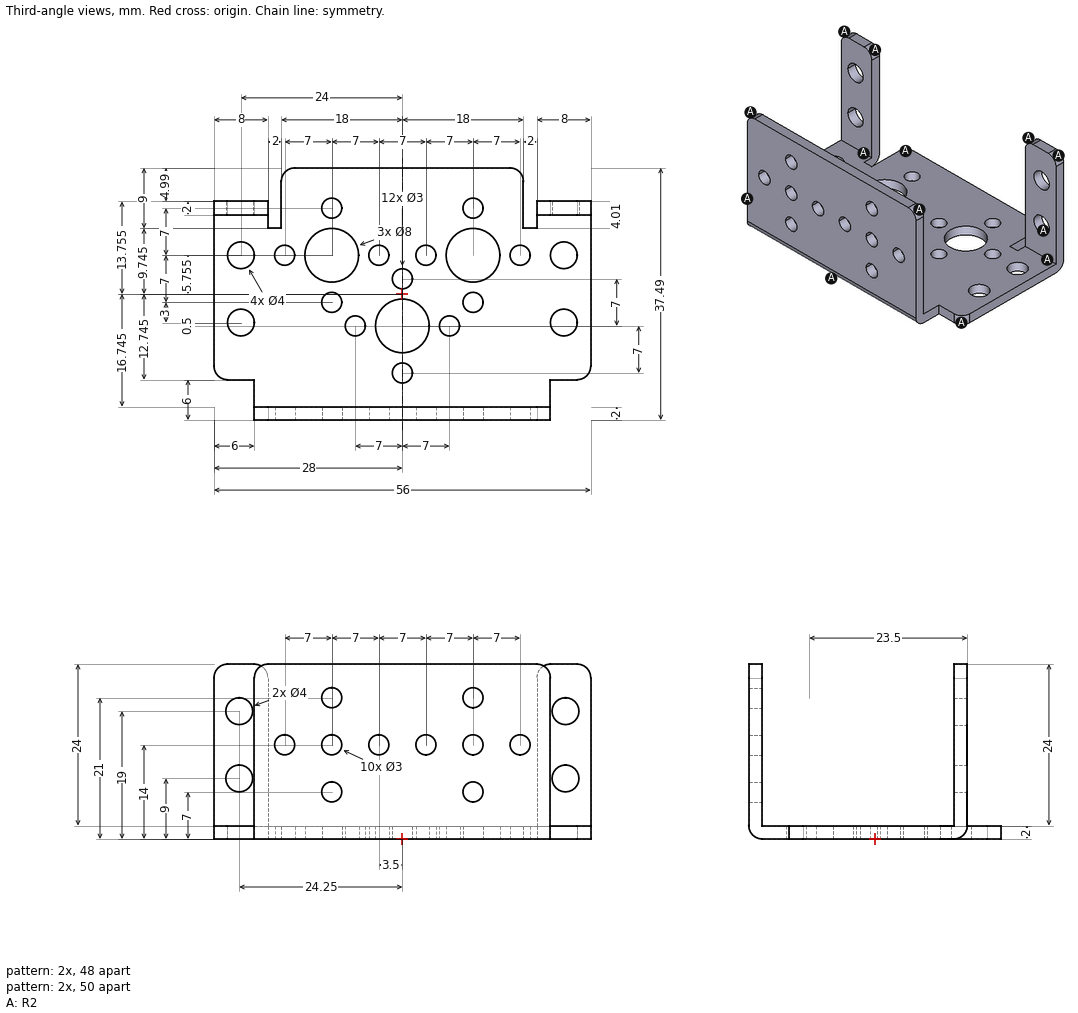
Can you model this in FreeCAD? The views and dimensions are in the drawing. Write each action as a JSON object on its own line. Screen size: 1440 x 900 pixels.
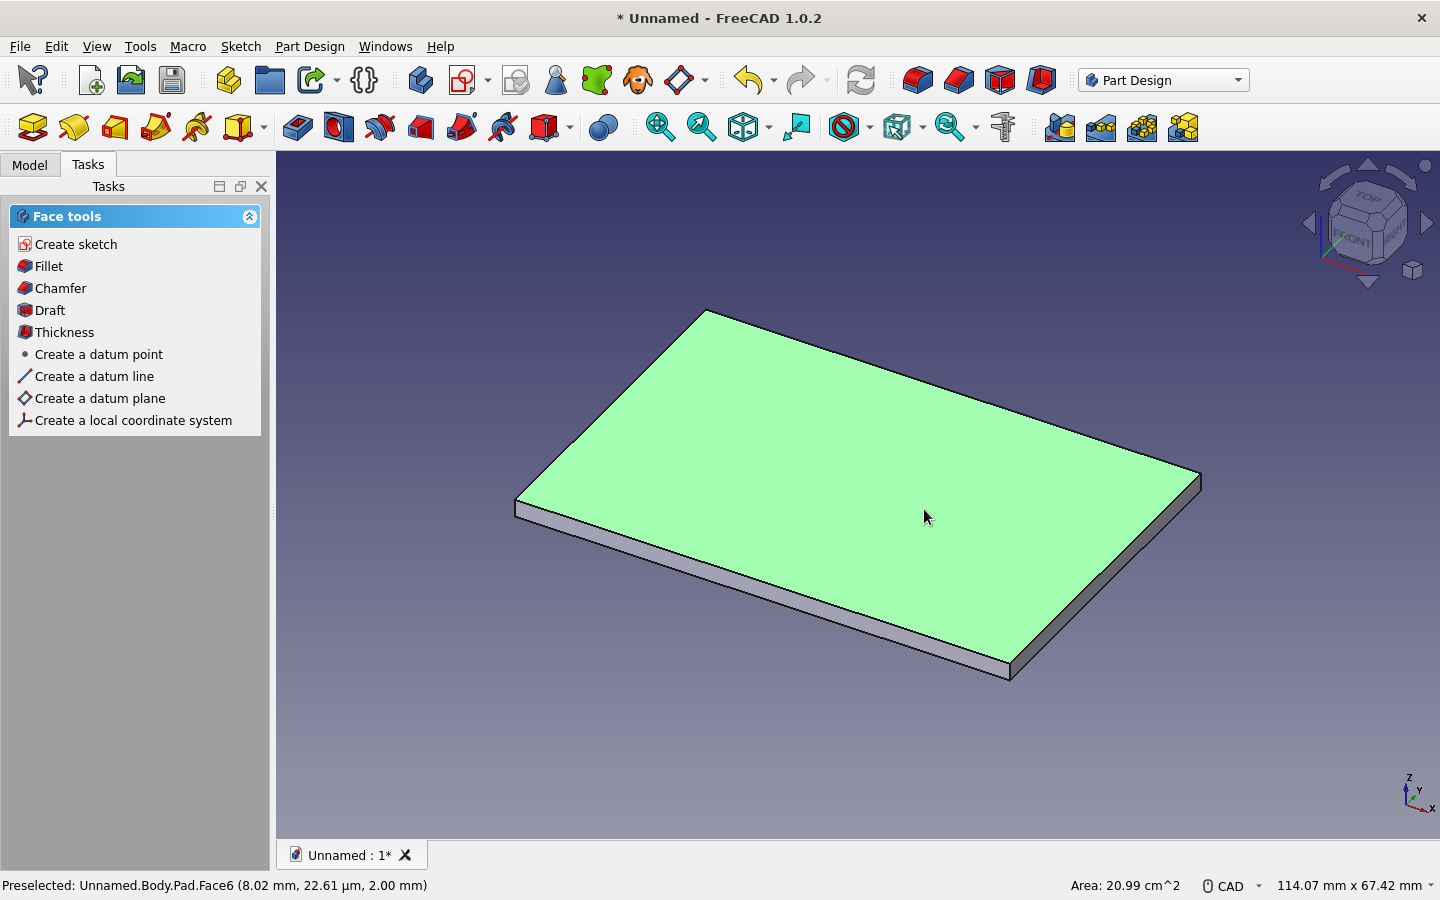
{"action": "left_click", "coordinate": [462, 80]}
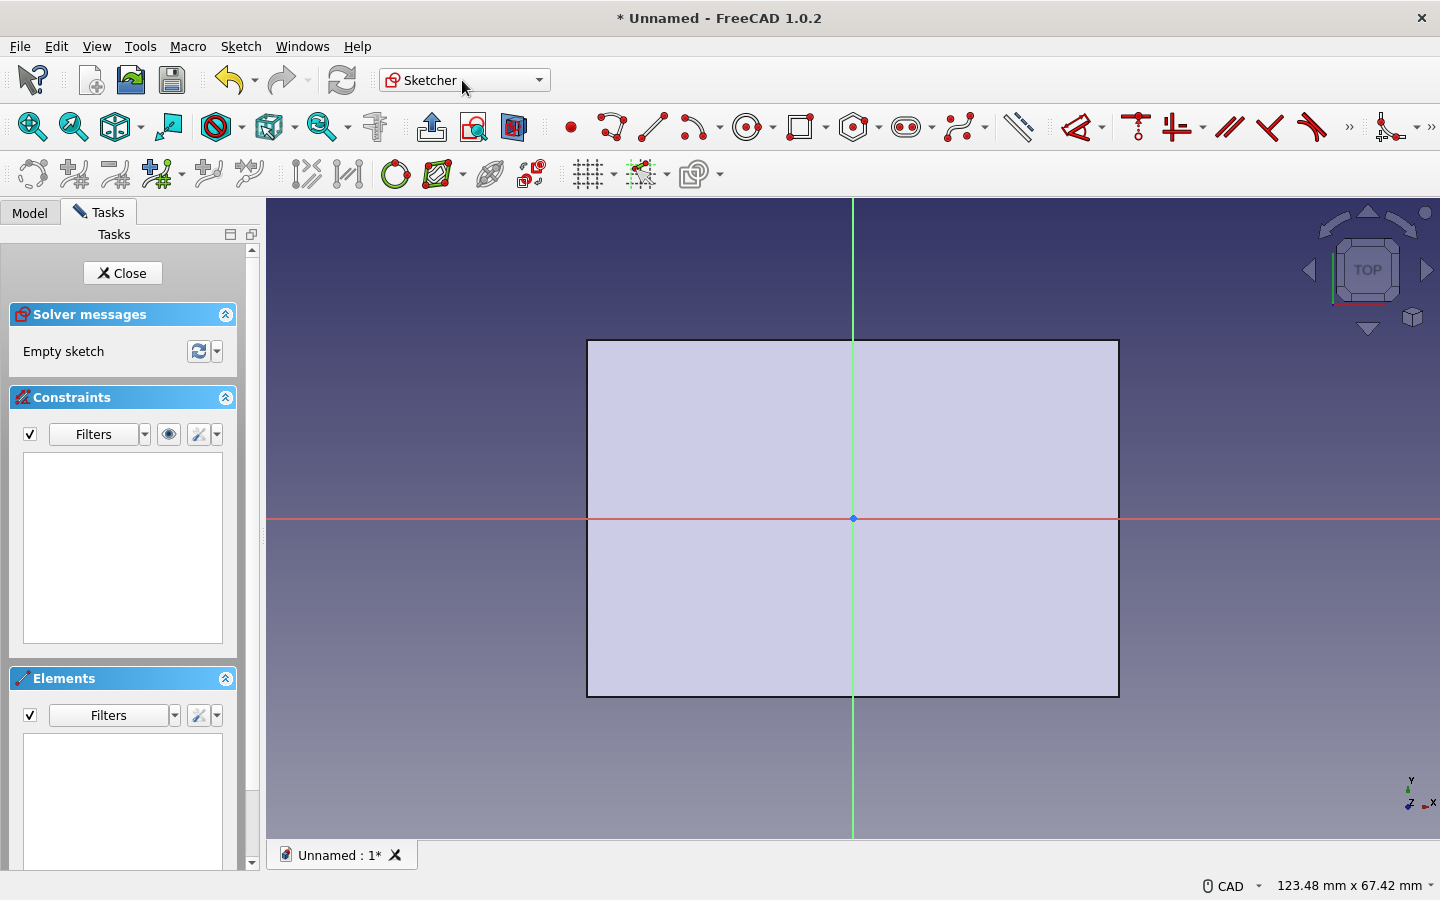
{"action": "key", "text": "g r"}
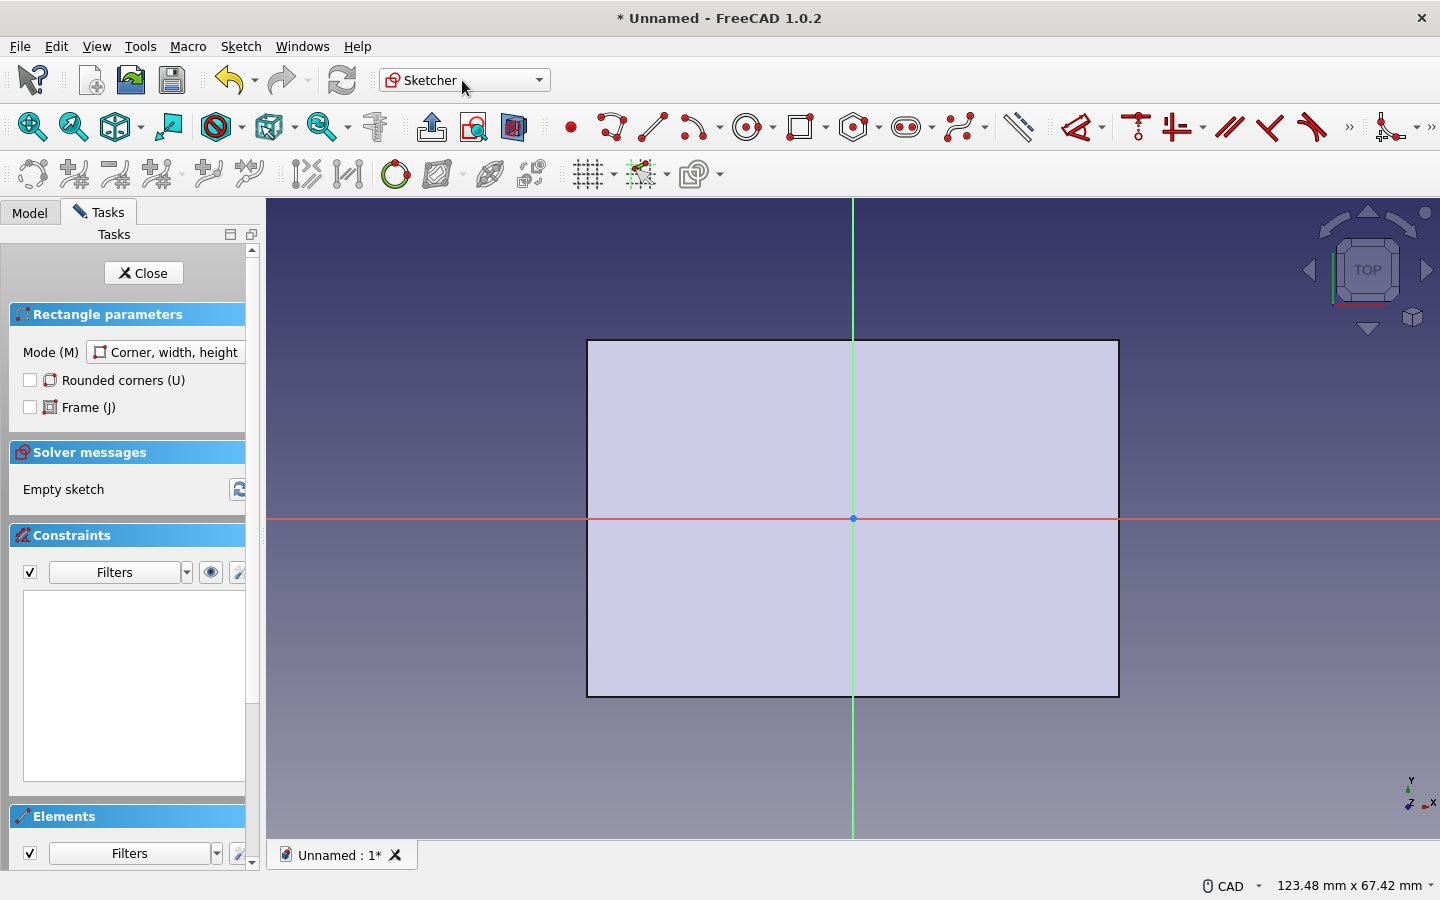
{"action": "left_click", "coordinate": [587, 678]}
{"action": "mouse_move", "coordinate": [1119, 697]}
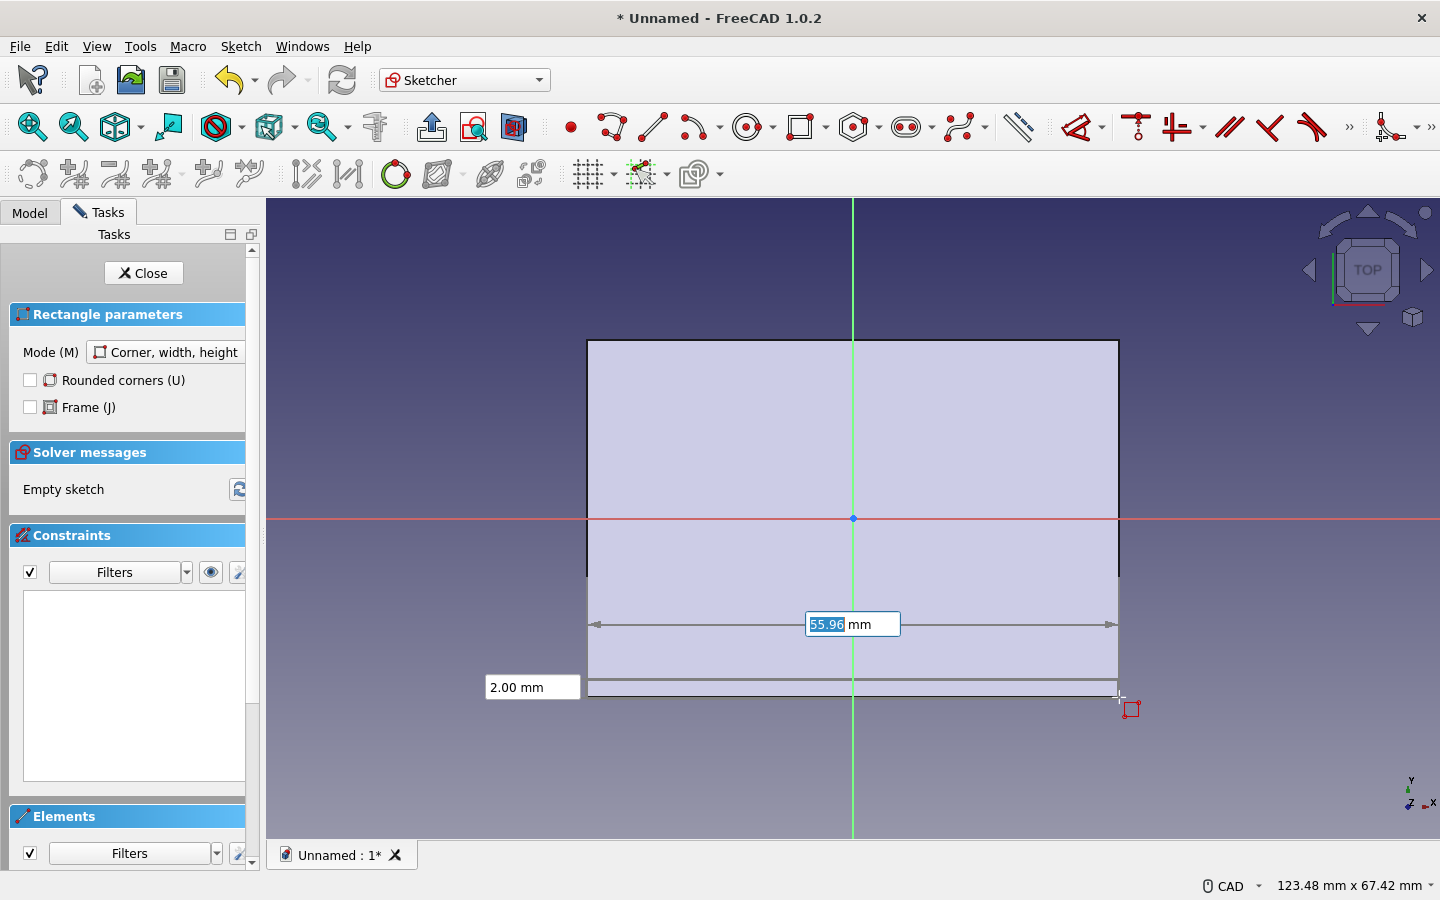
{"action": "type", "text": "56"}
{"action": "key", "text": "Tab"}
{"action": "type", "text": "2"}
{"action": "key", "text": "Return"}
{"action": "key", "text": "Escape"}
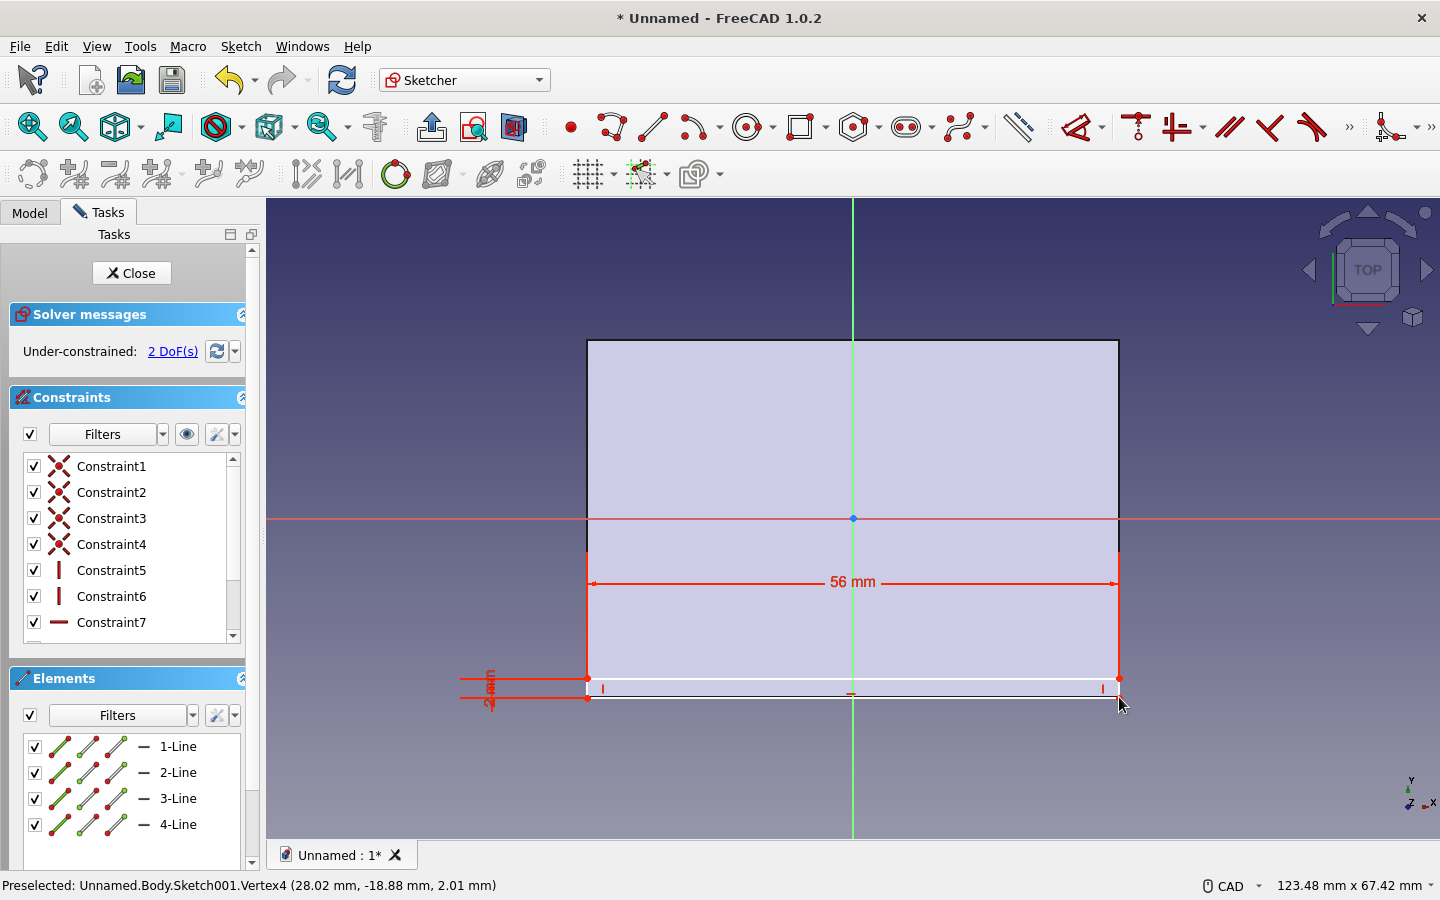
{"action": "left_click", "coordinate": [587, 679]}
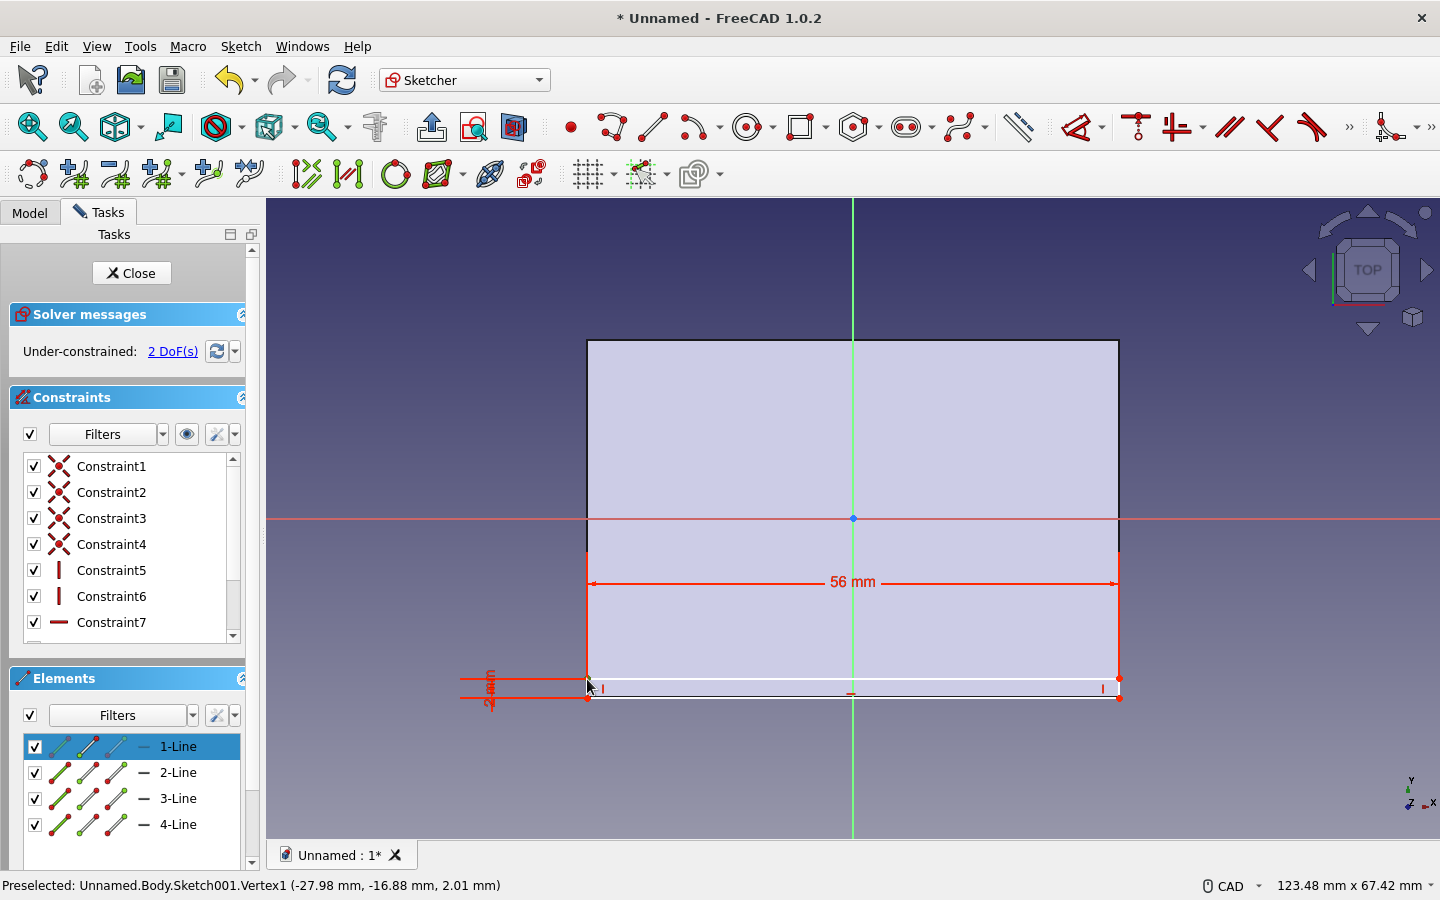
{"action": "left_click", "coordinate": [1102, 128]}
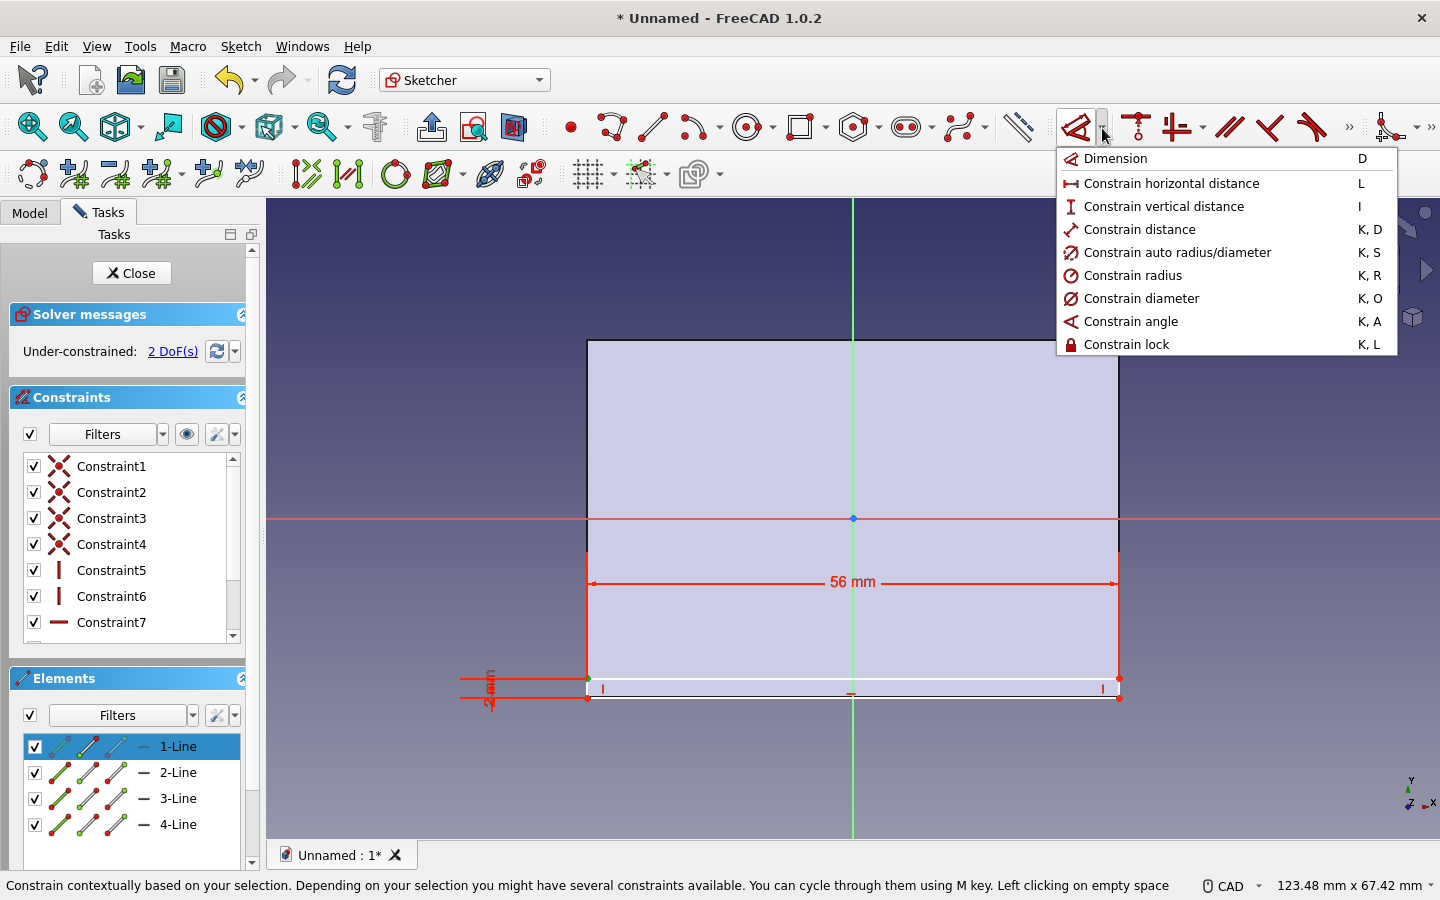
{"action": "left_click", "coordinate": [1227, 184]}